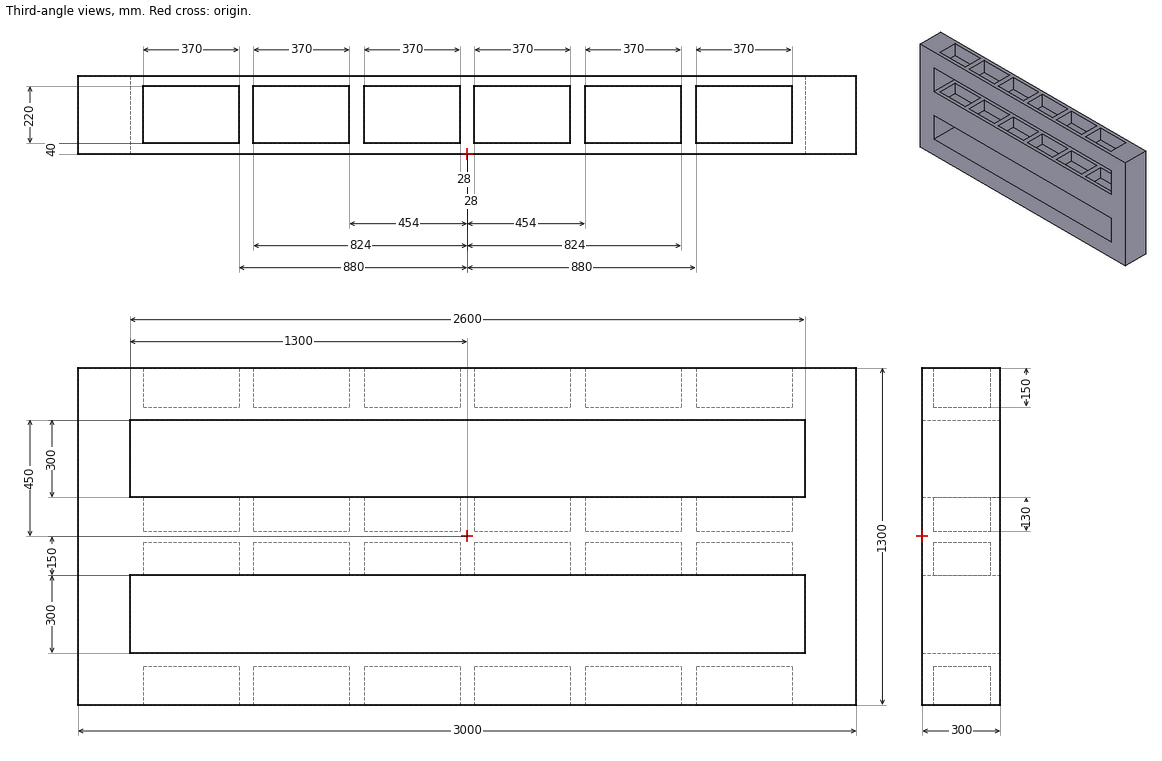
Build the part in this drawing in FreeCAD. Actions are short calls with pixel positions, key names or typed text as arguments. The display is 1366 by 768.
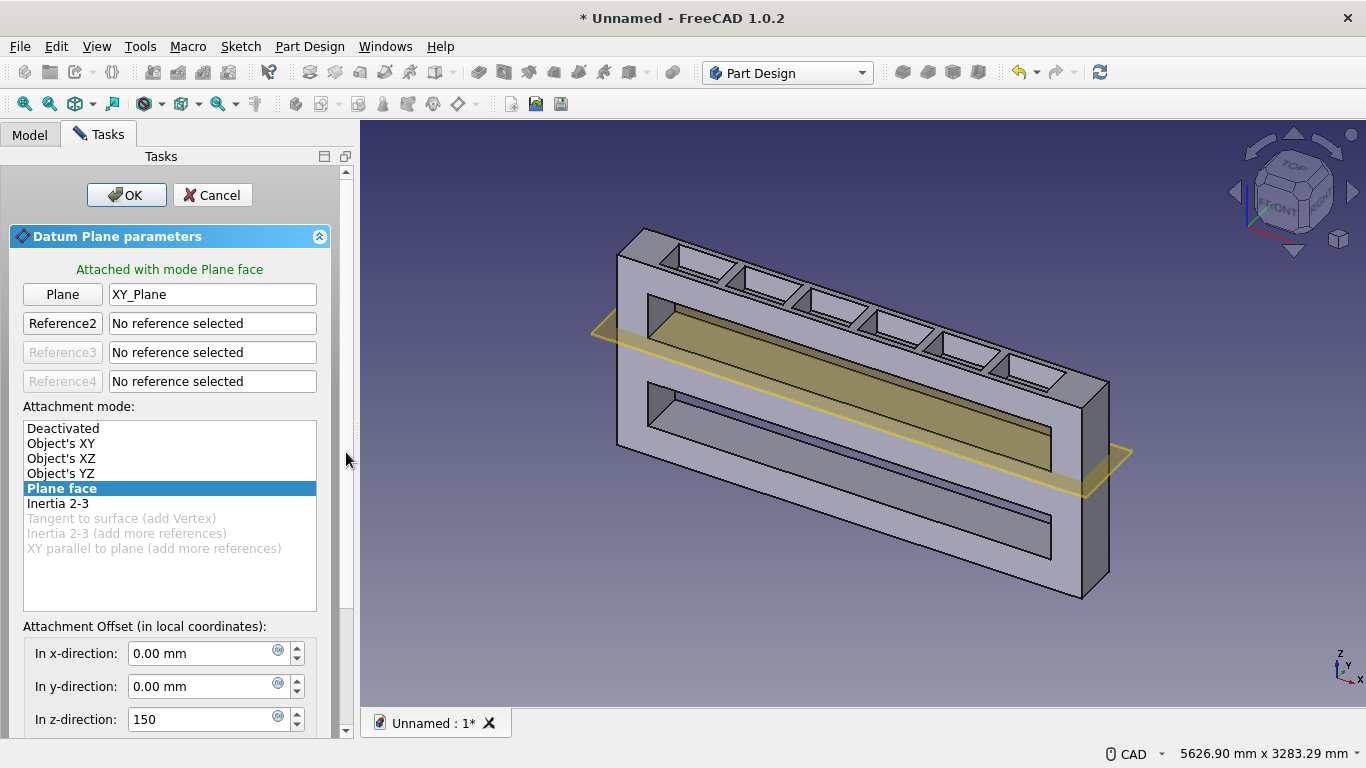
click(127, 195)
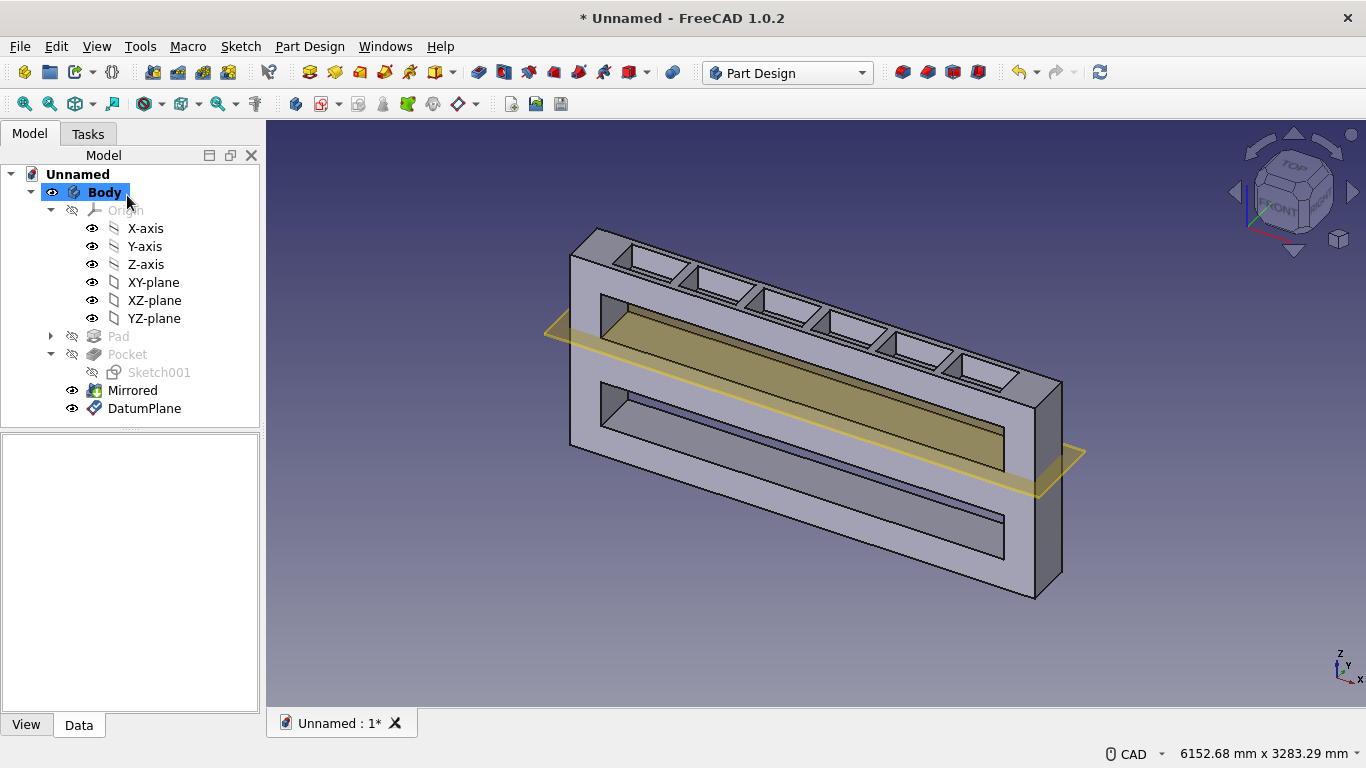
click(117, 408)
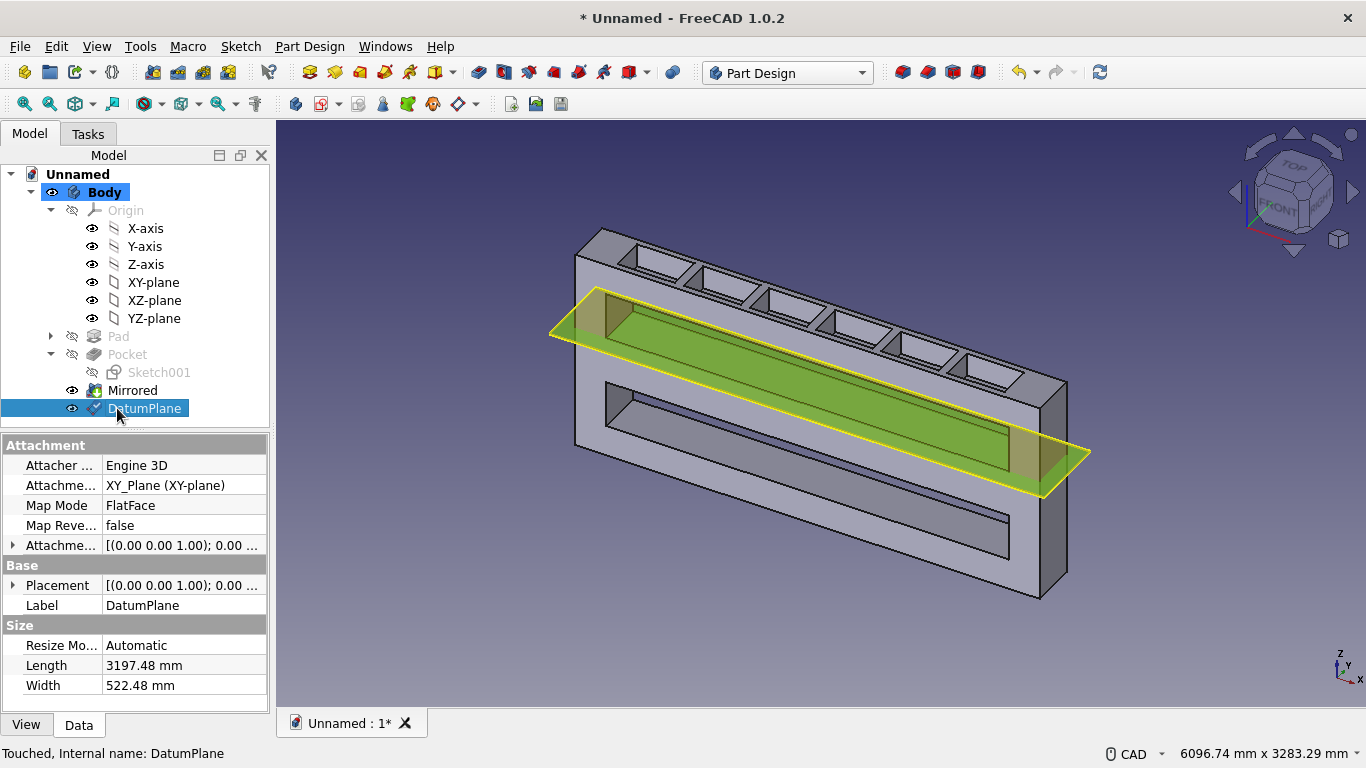
click(320, 104)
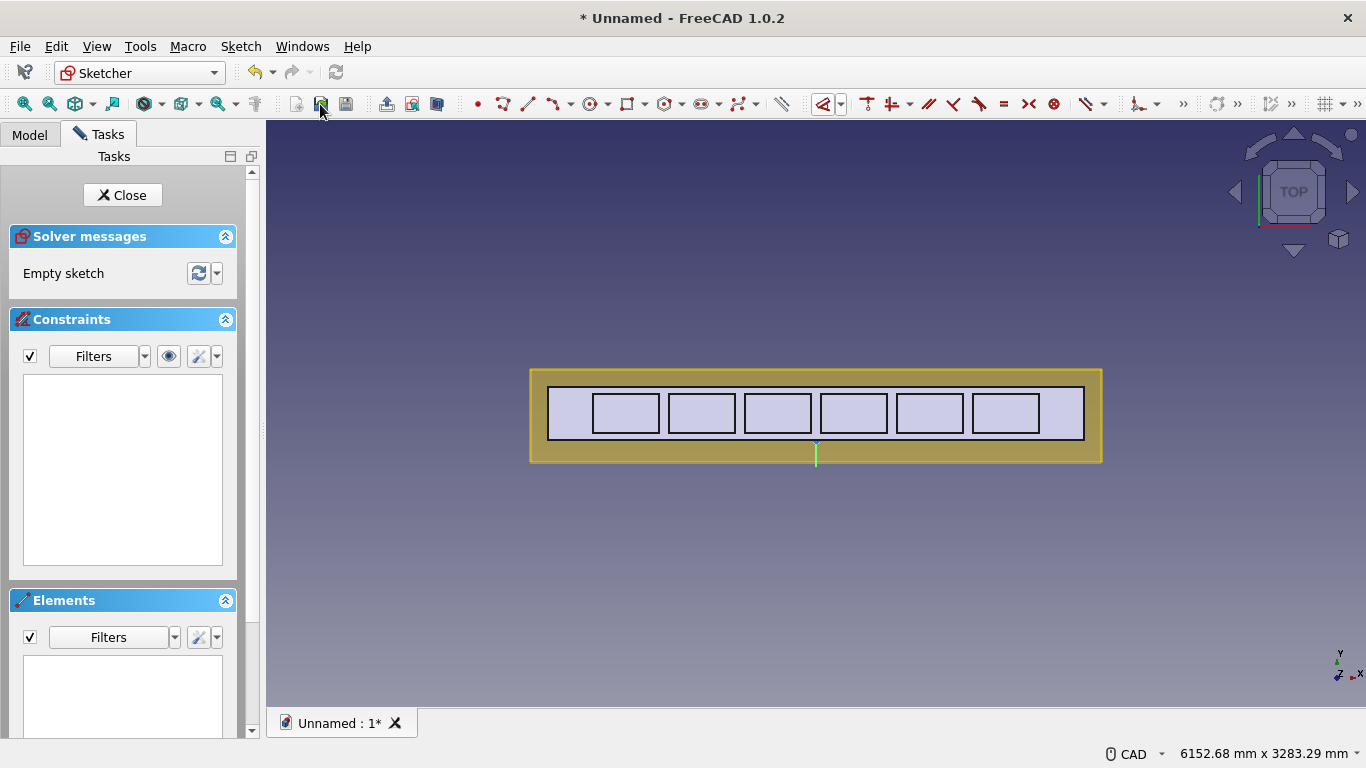
key(q)
key(s)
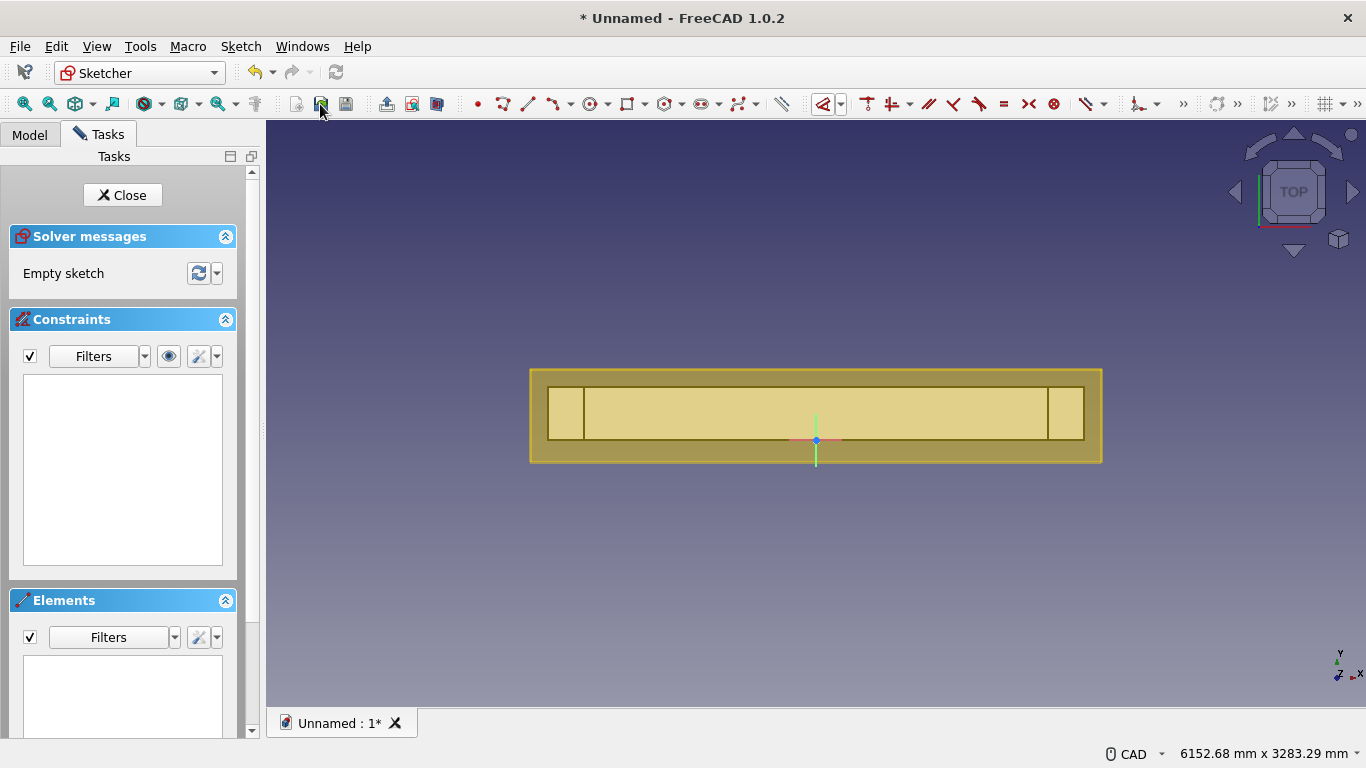
scroll(955, 424, up, 2)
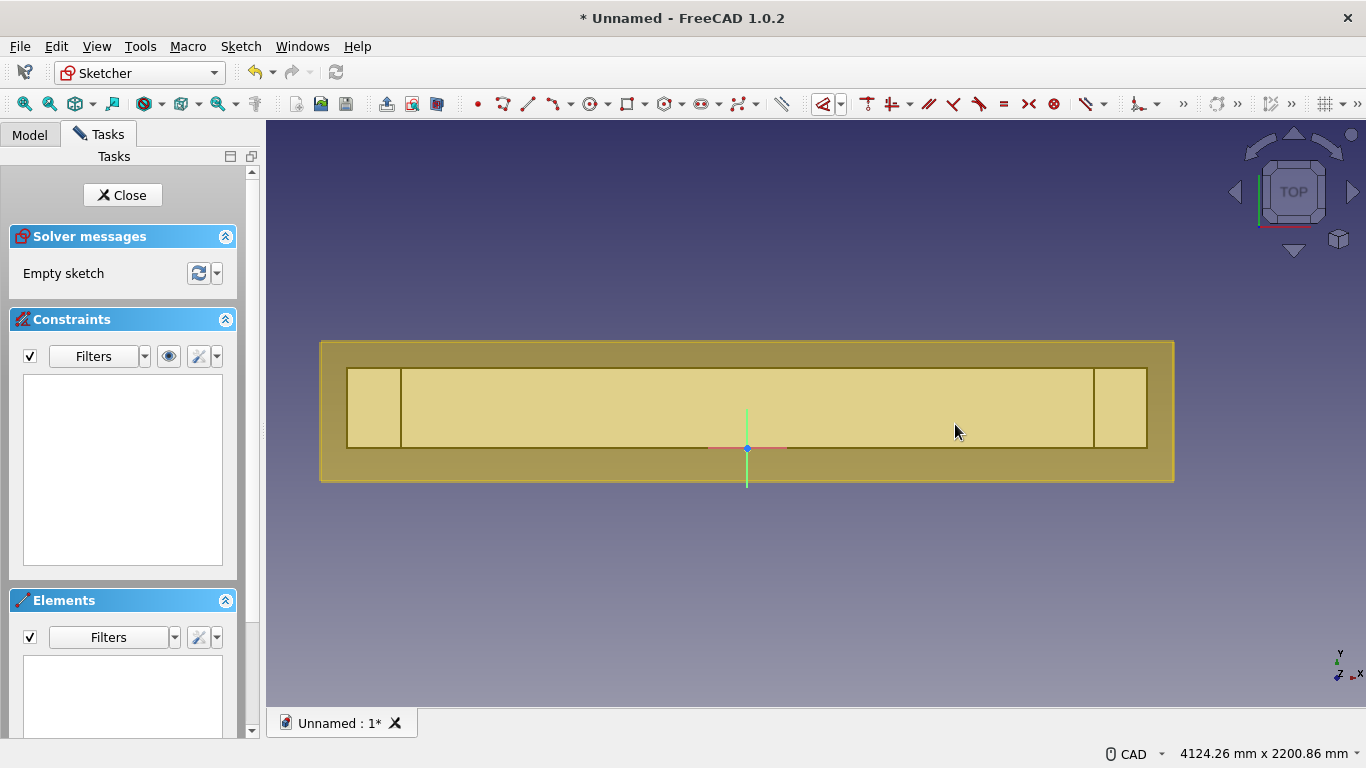
key(g)
key(r)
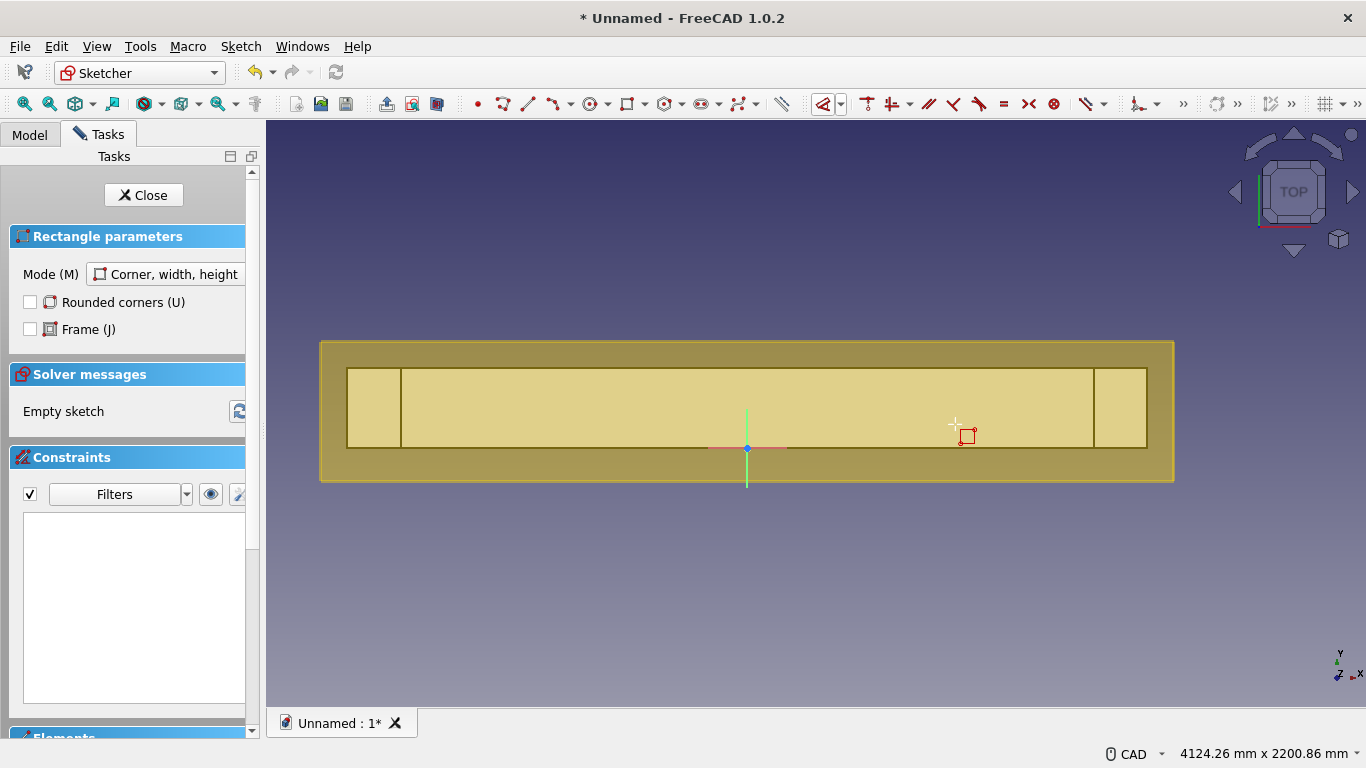
click(414, 379)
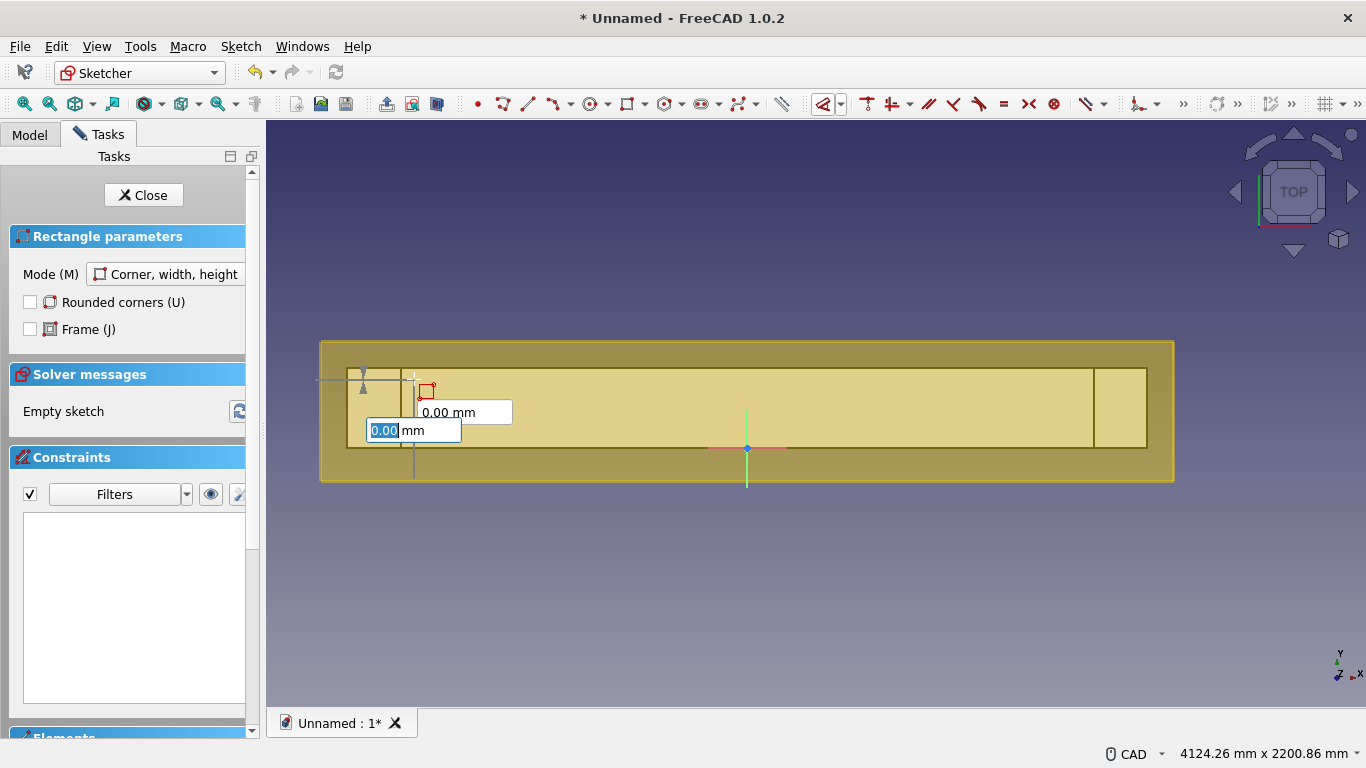
scroll(513, 437, up, 2)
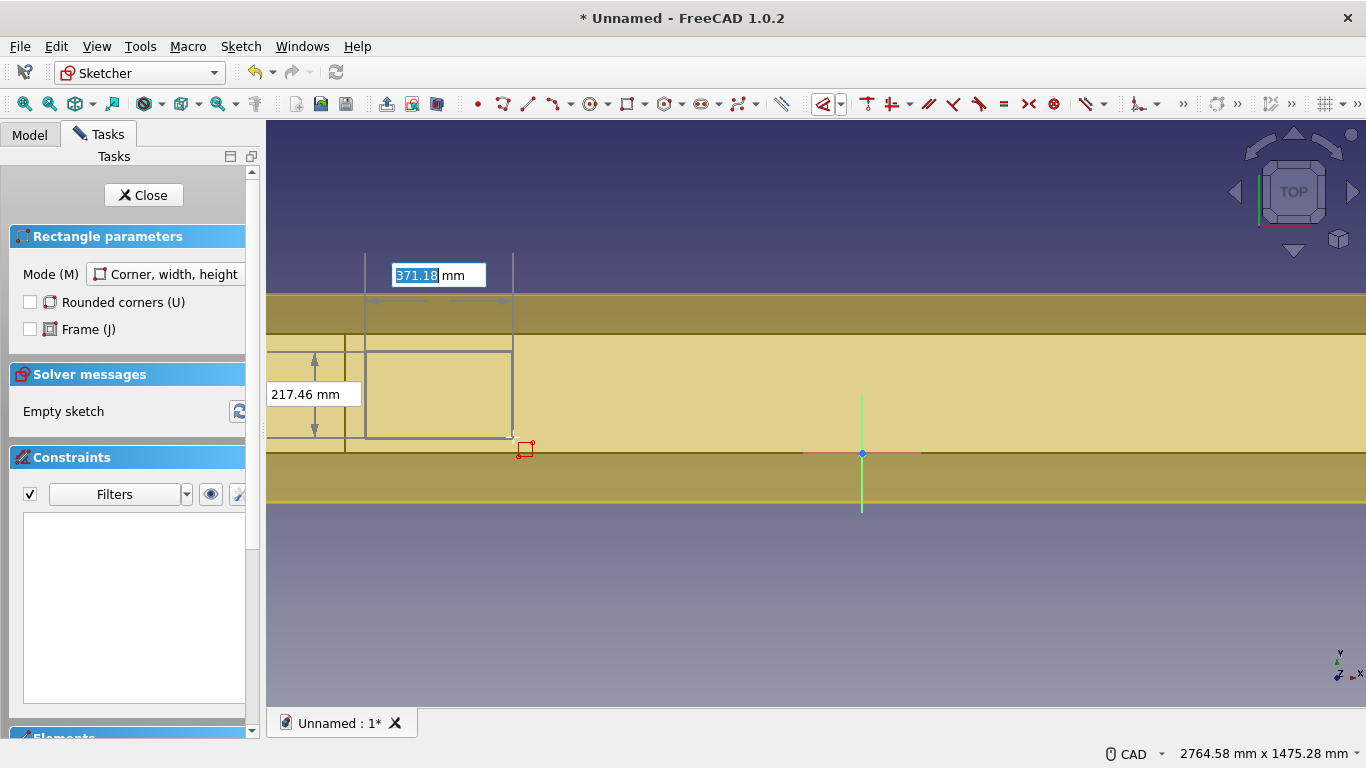
click(512, 437)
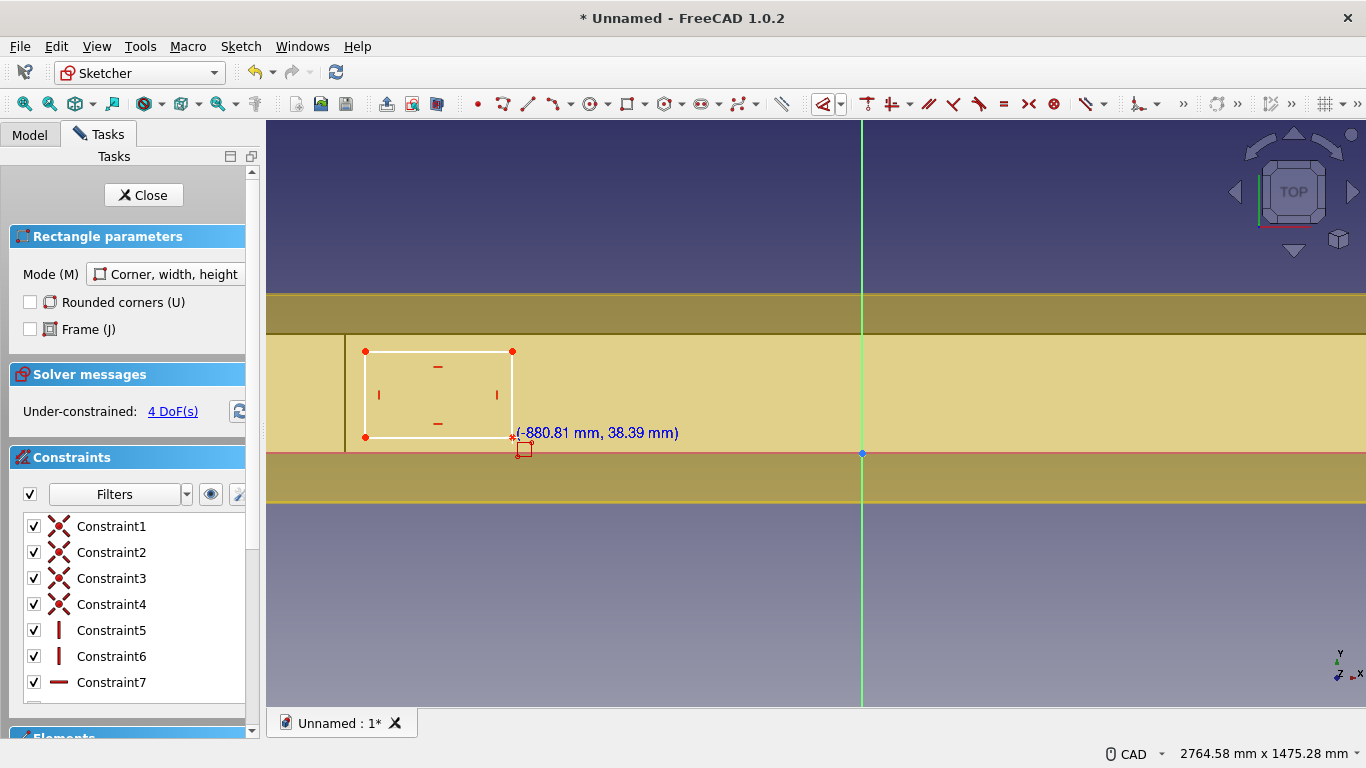
click(535, 350)
click(682, 437)